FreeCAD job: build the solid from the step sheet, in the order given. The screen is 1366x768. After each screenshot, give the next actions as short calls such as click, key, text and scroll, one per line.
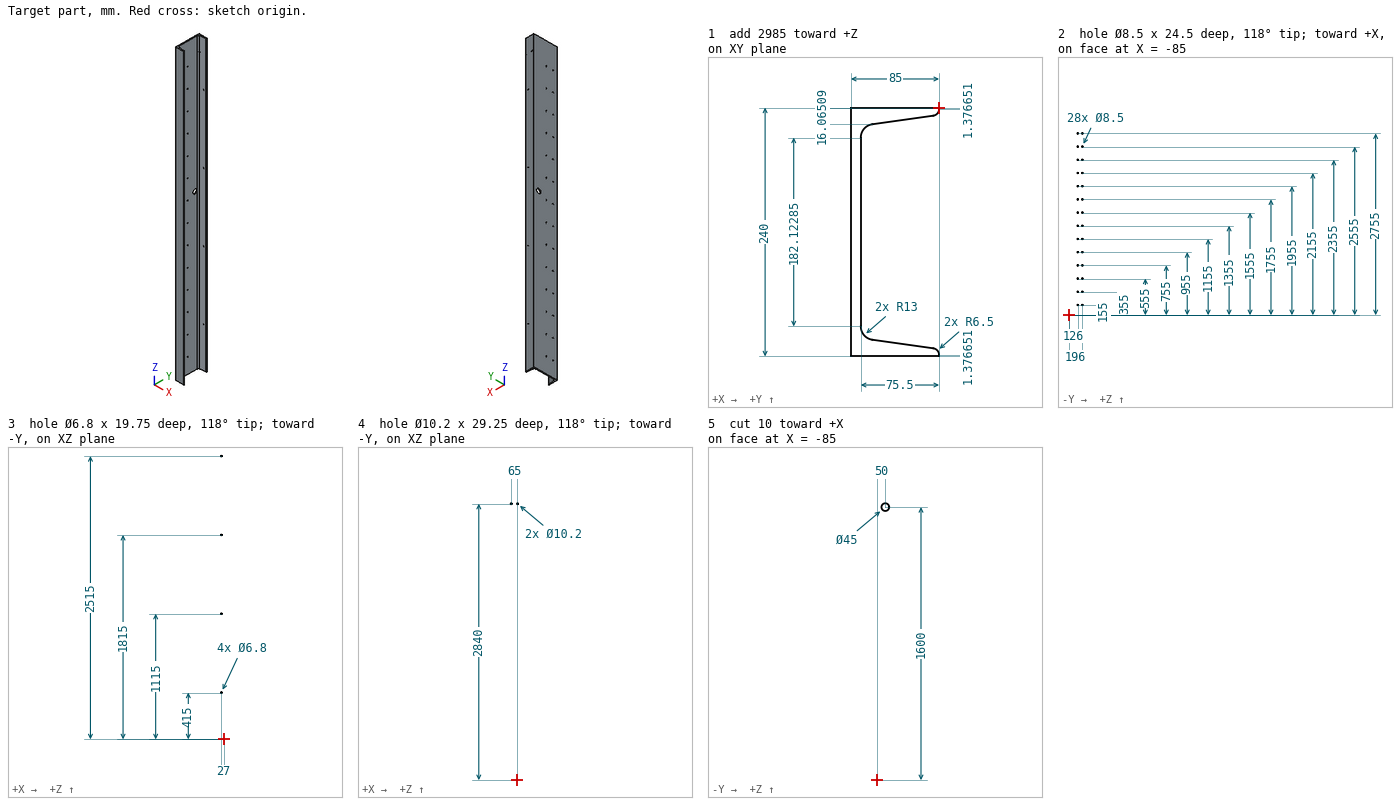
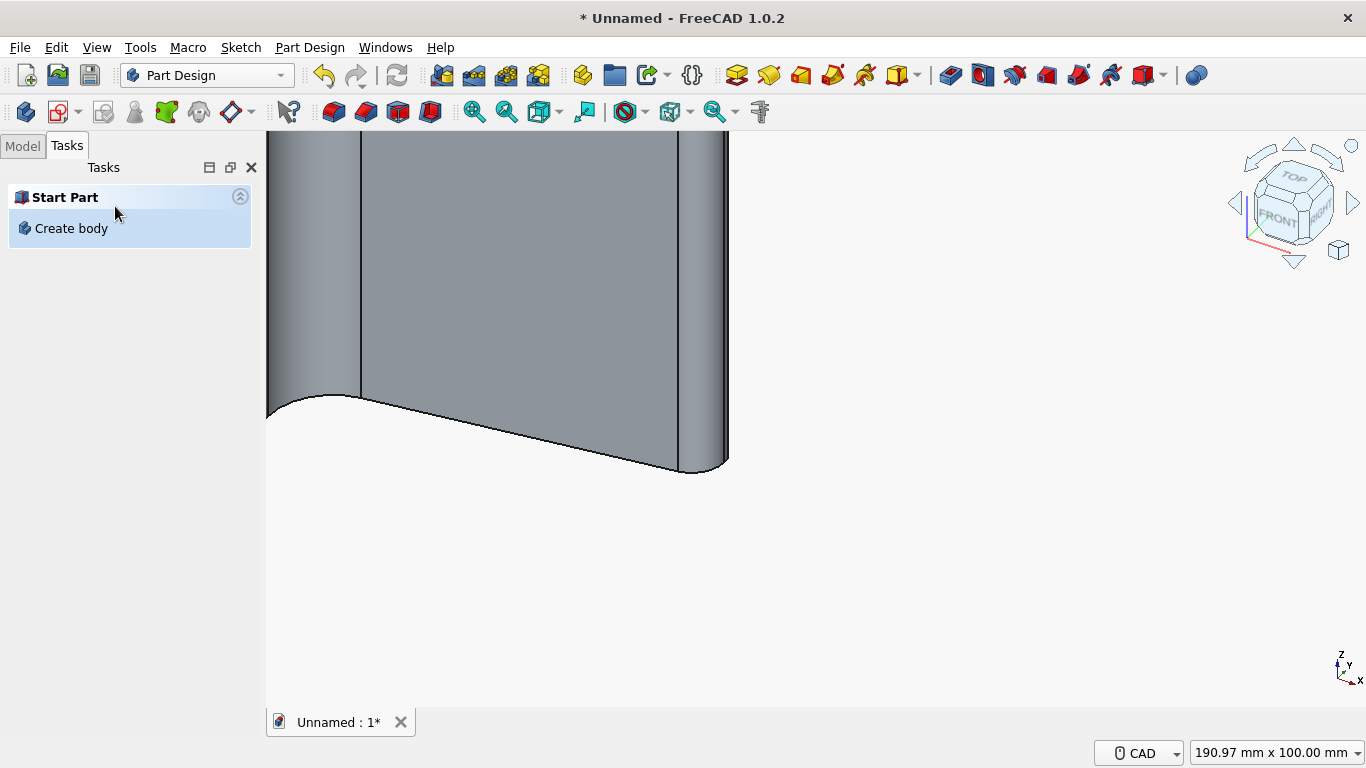
click(476, 112)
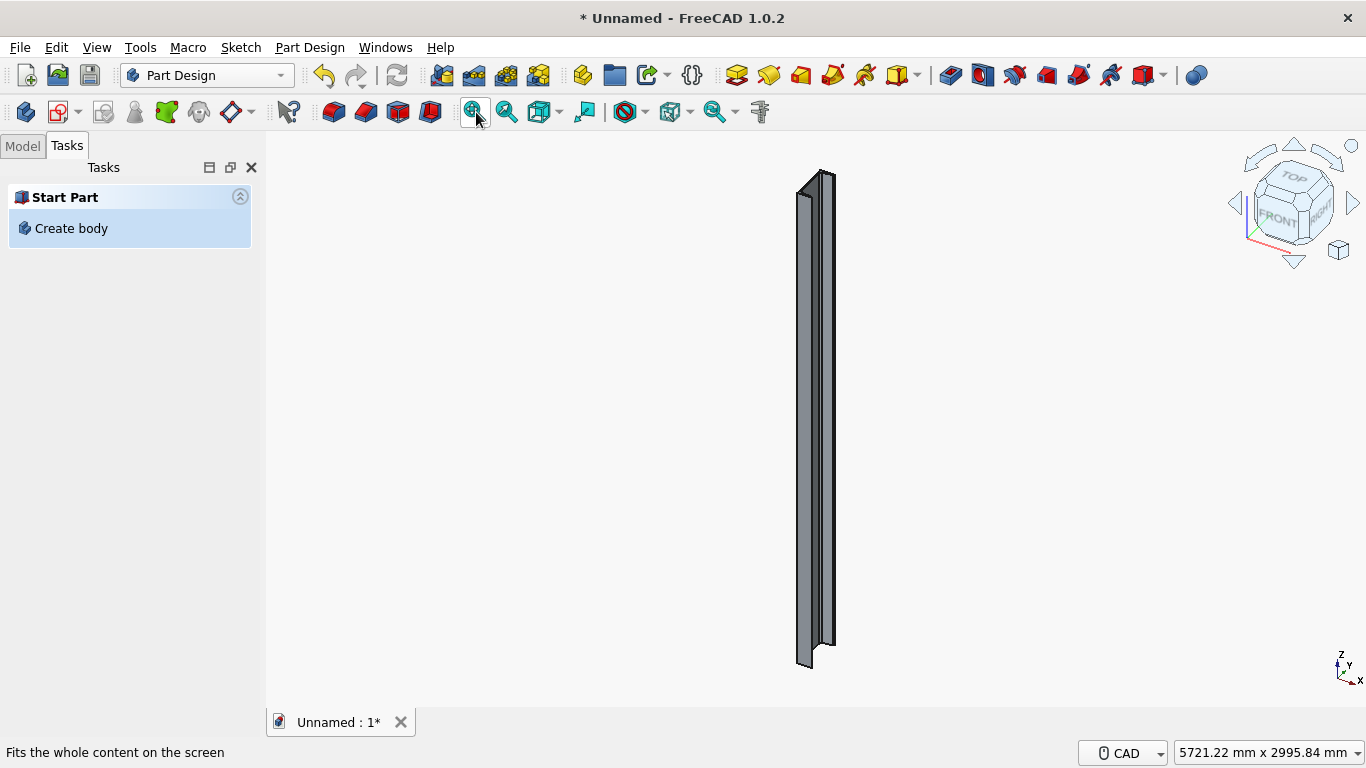
key(6)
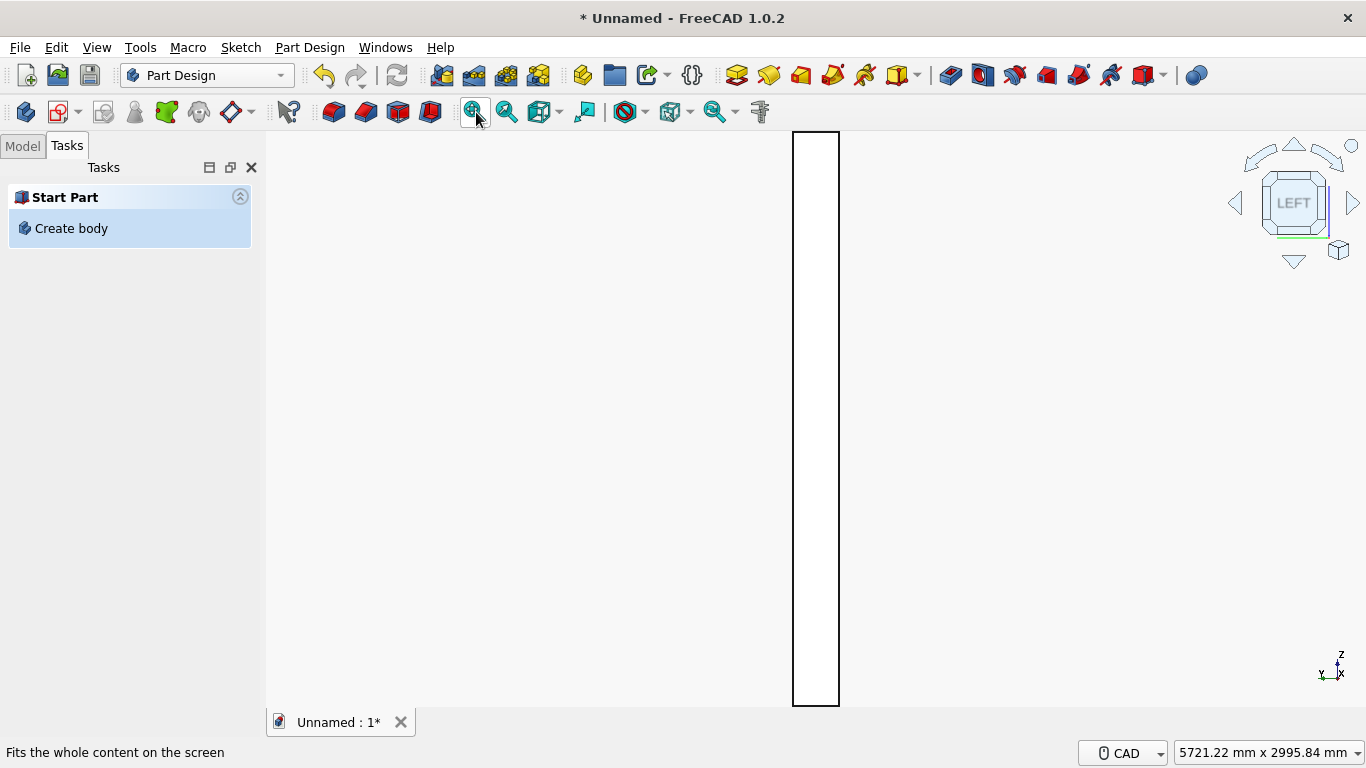
click(816, 172)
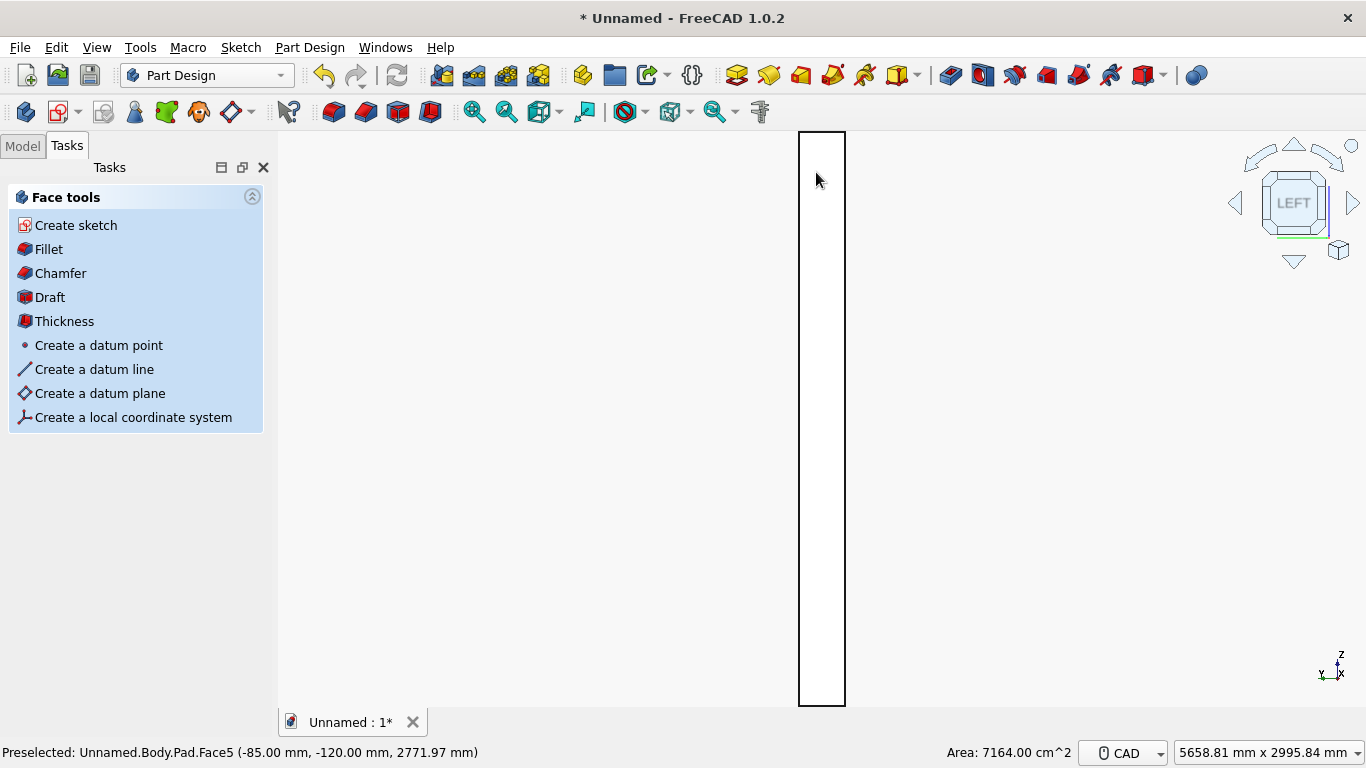
click(58, 112)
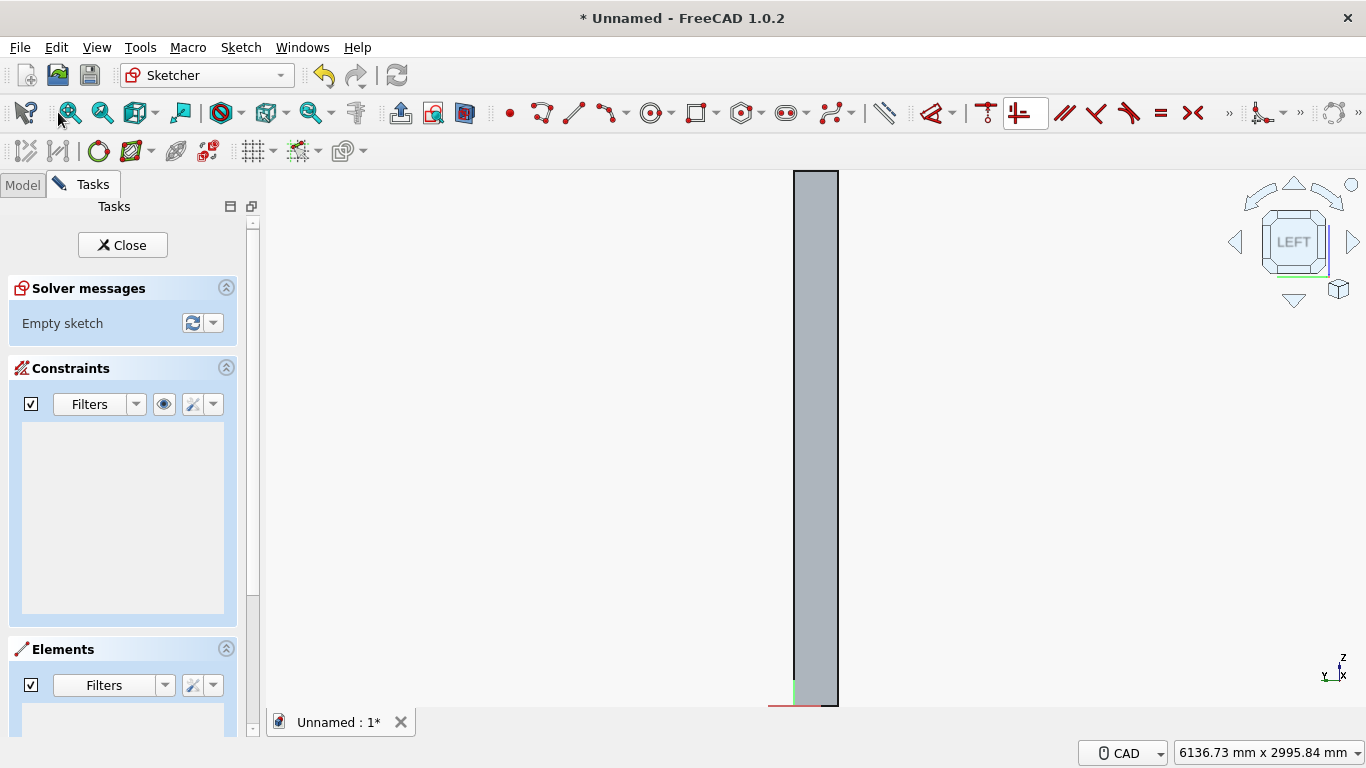
scroll(615, 397, down, 2)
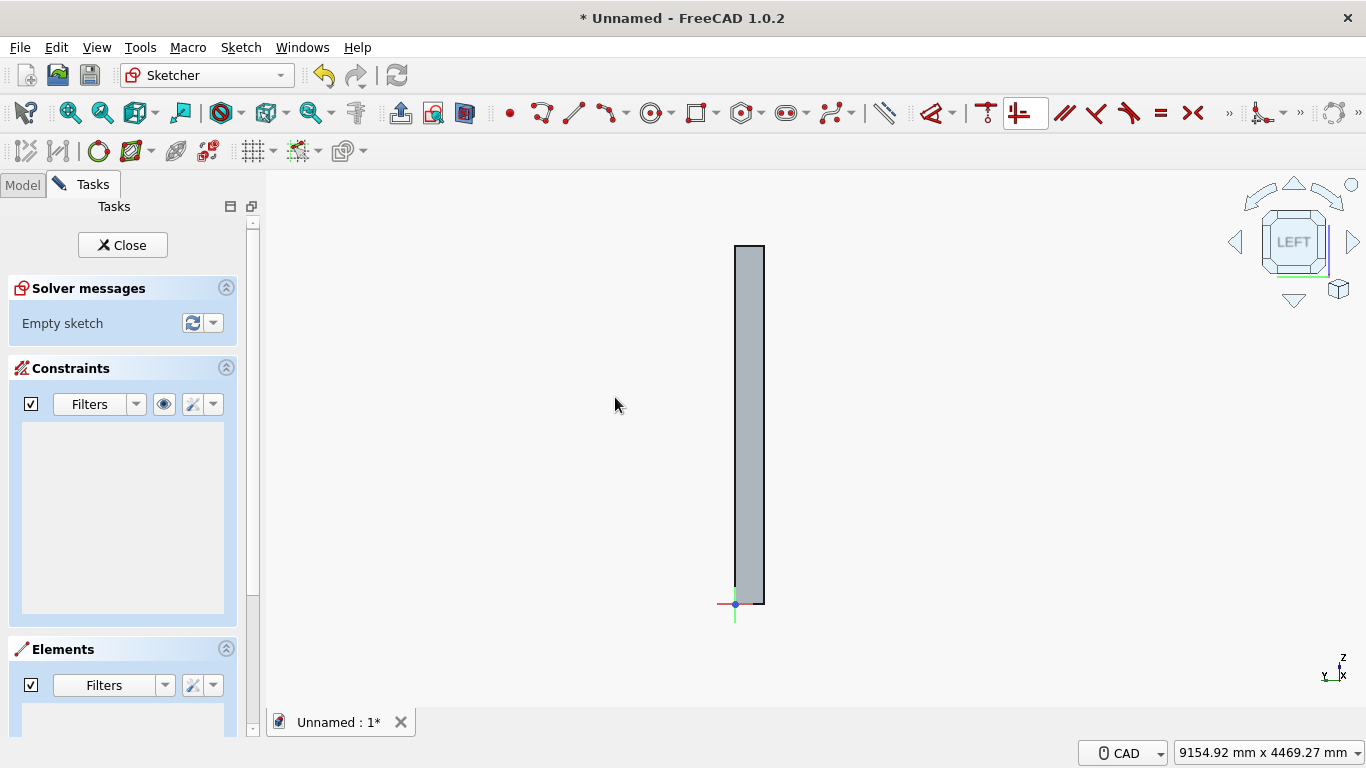
click(652, 114)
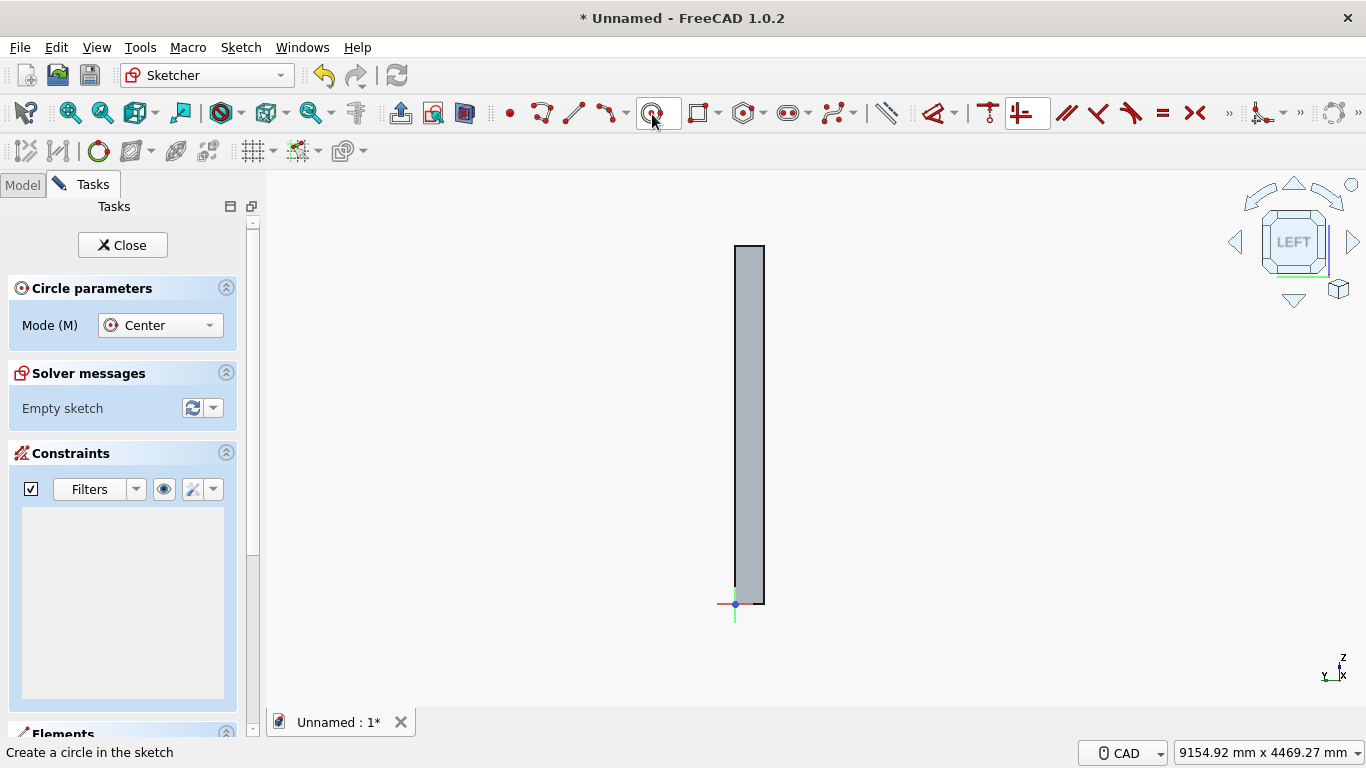
scroll(751, 586, up, 19)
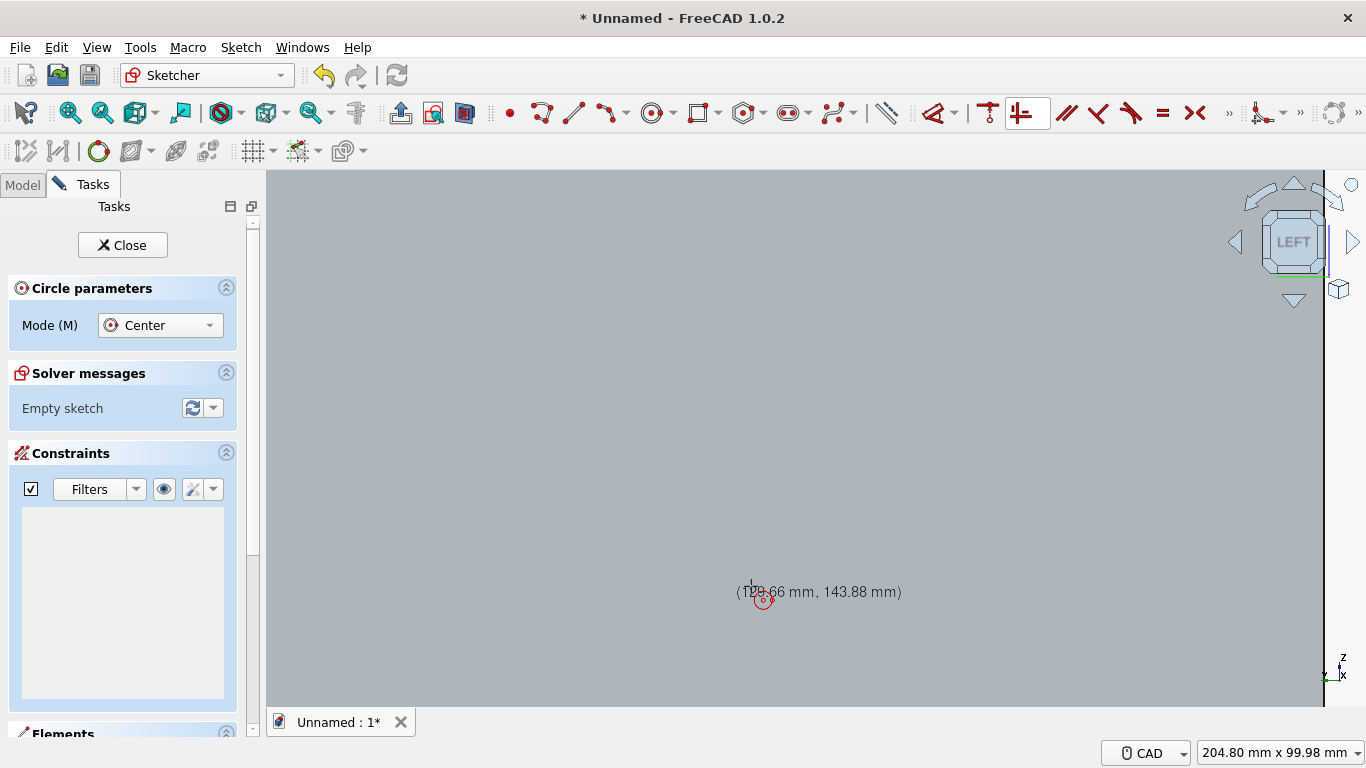
scroll(752, 621, down, 18)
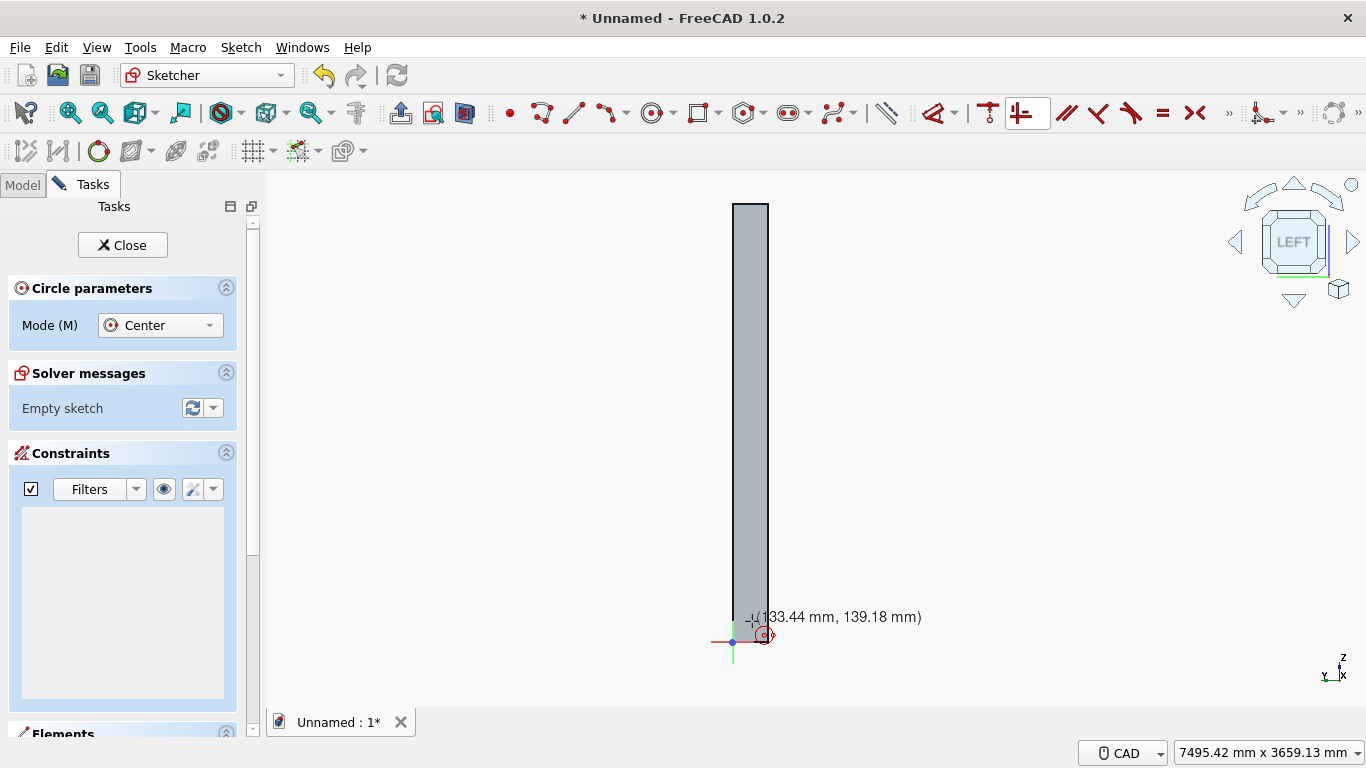
click(751, 620)
move(752, 619)